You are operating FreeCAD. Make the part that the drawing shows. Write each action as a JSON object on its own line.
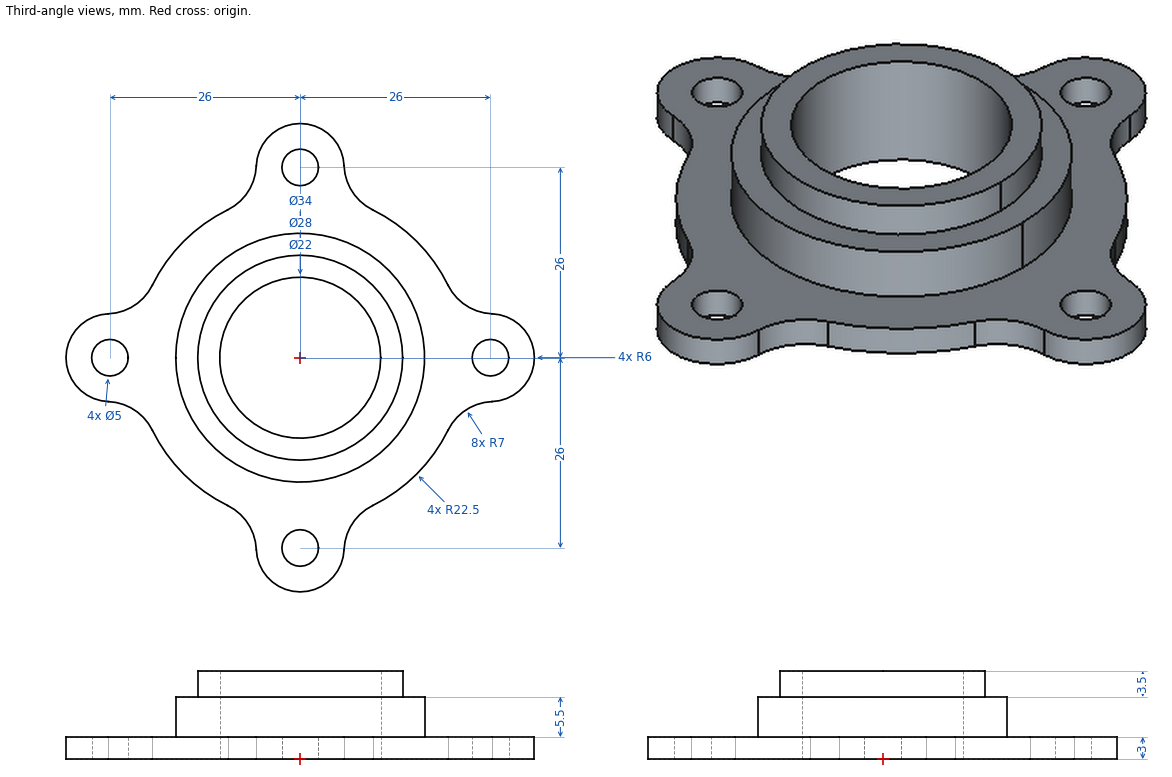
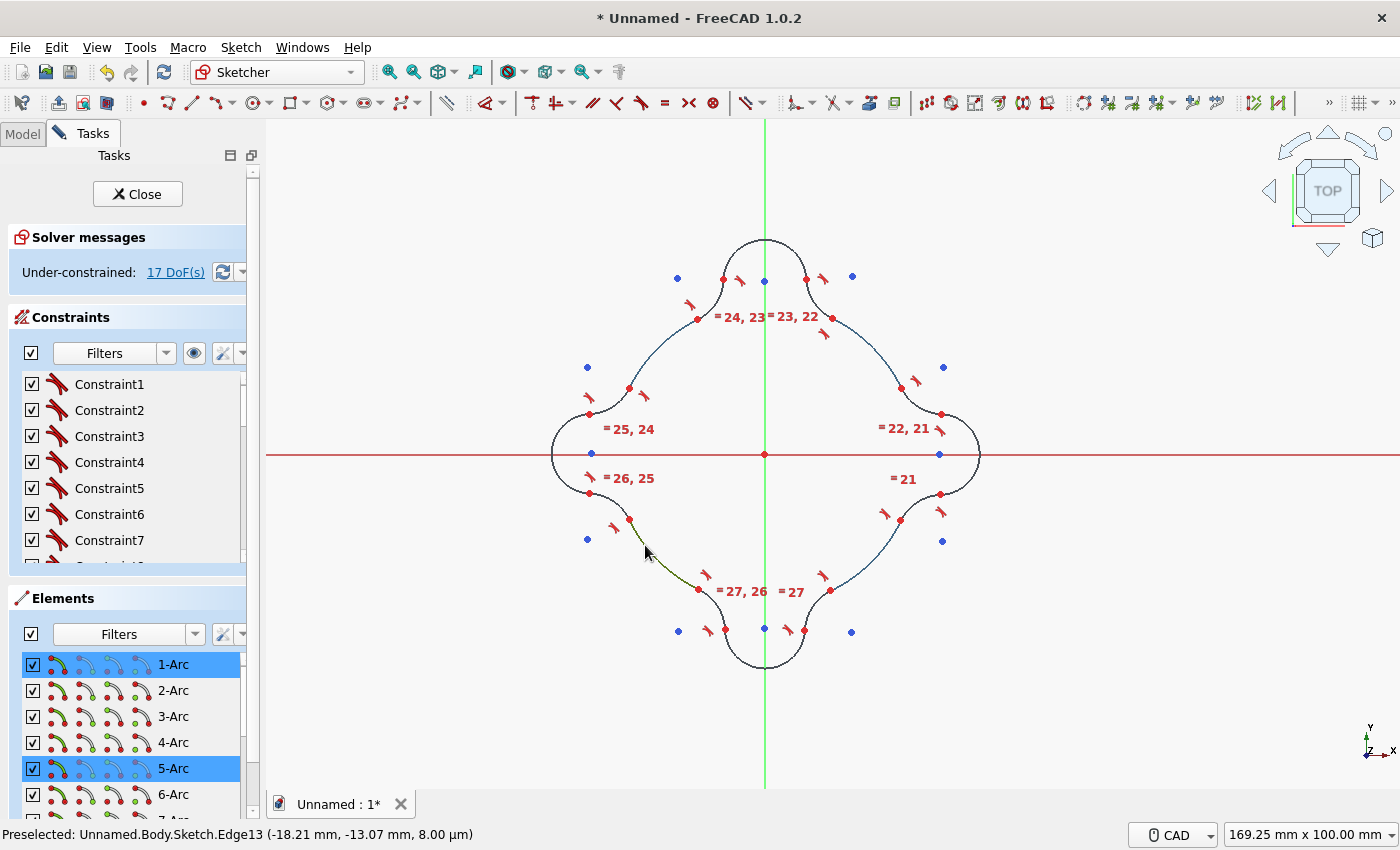
{"action": "left_click", "coordinate": [666, 104]}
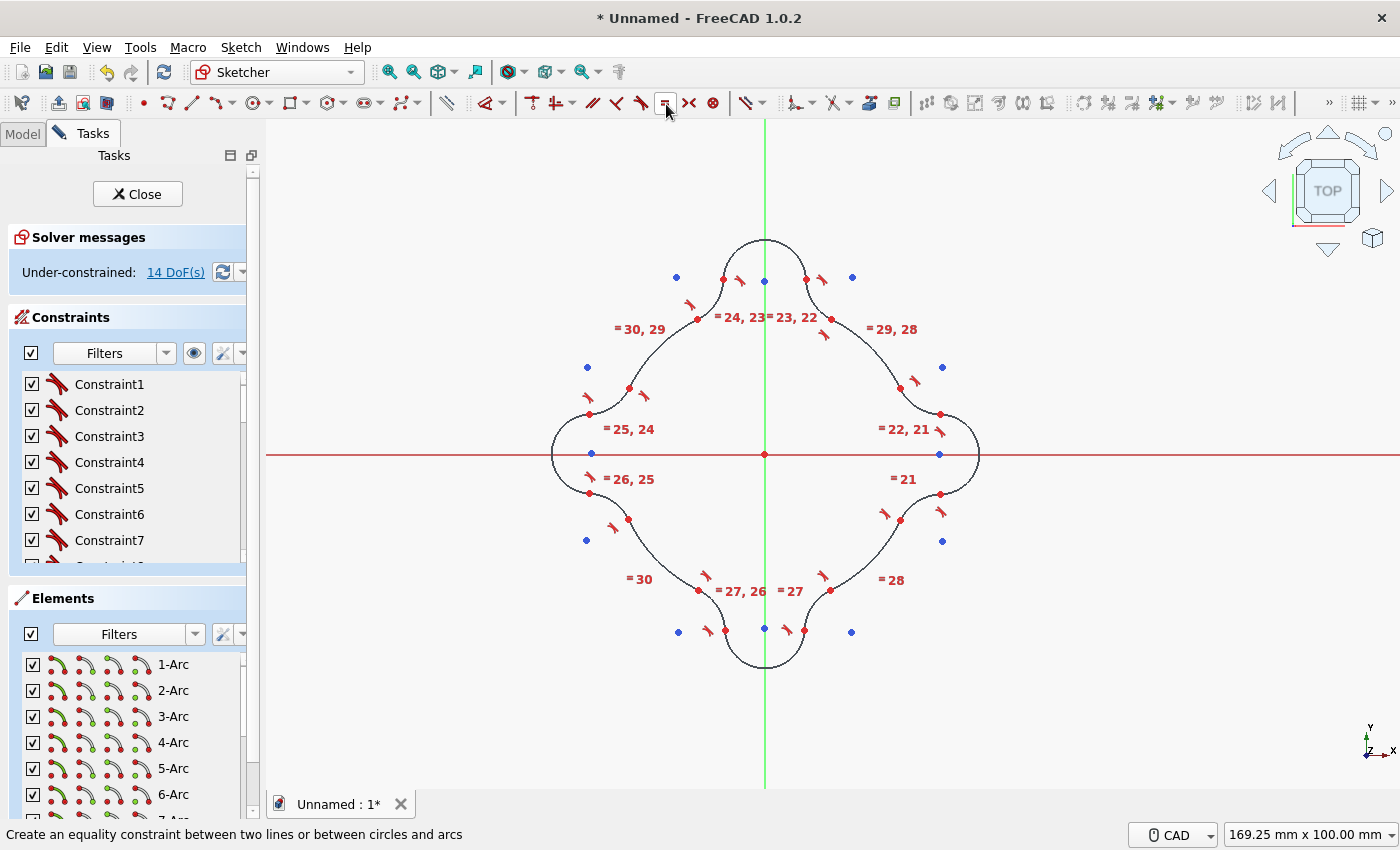
{"action": "left_click", "coordinate": [972, 478]}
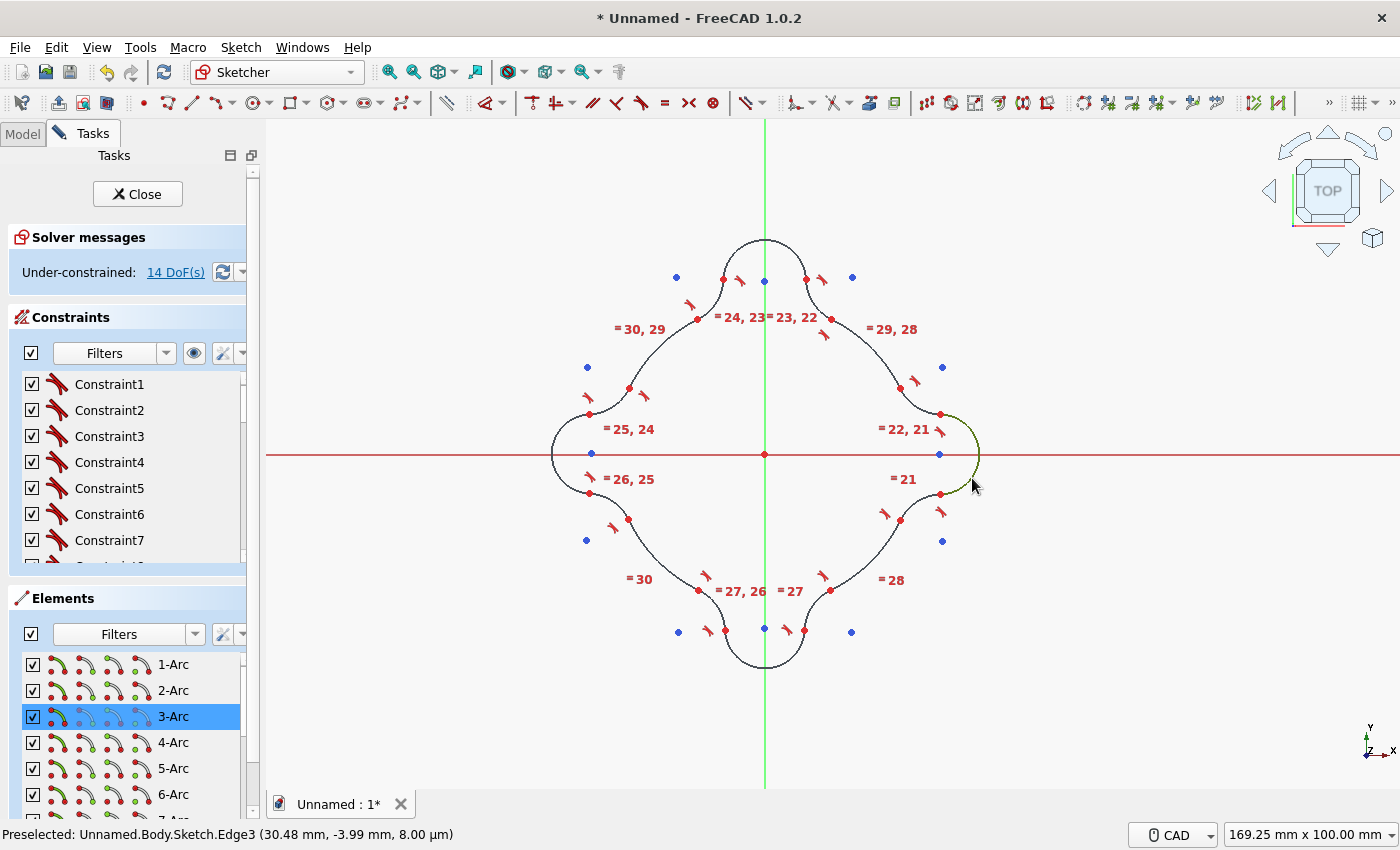
{"action": "left_click", "coordinate": [788, 248]}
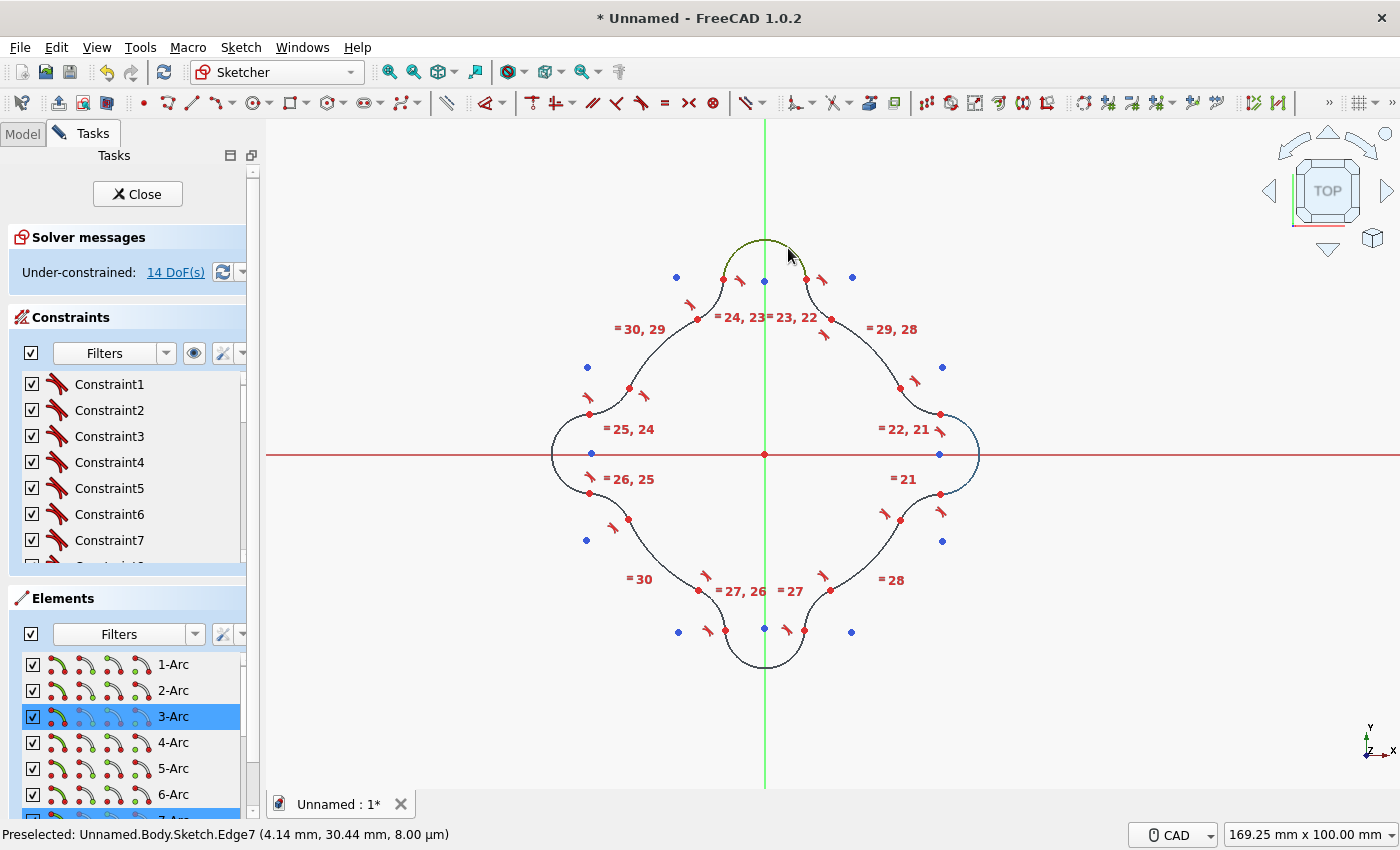
{"action": "left_click", "coordinate": [559, 431]}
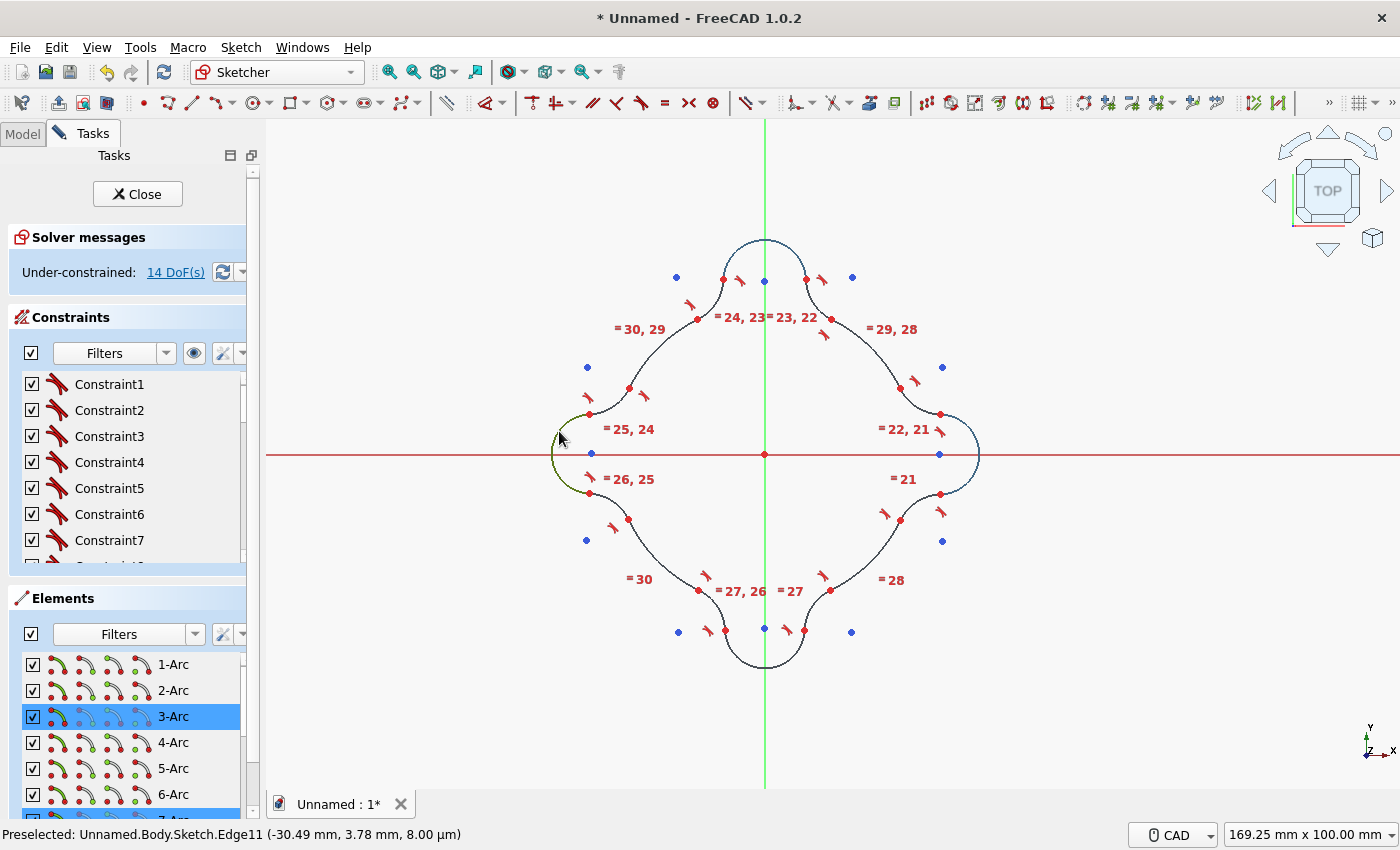
{"action": "left_click", "coordinate": [742, 661]}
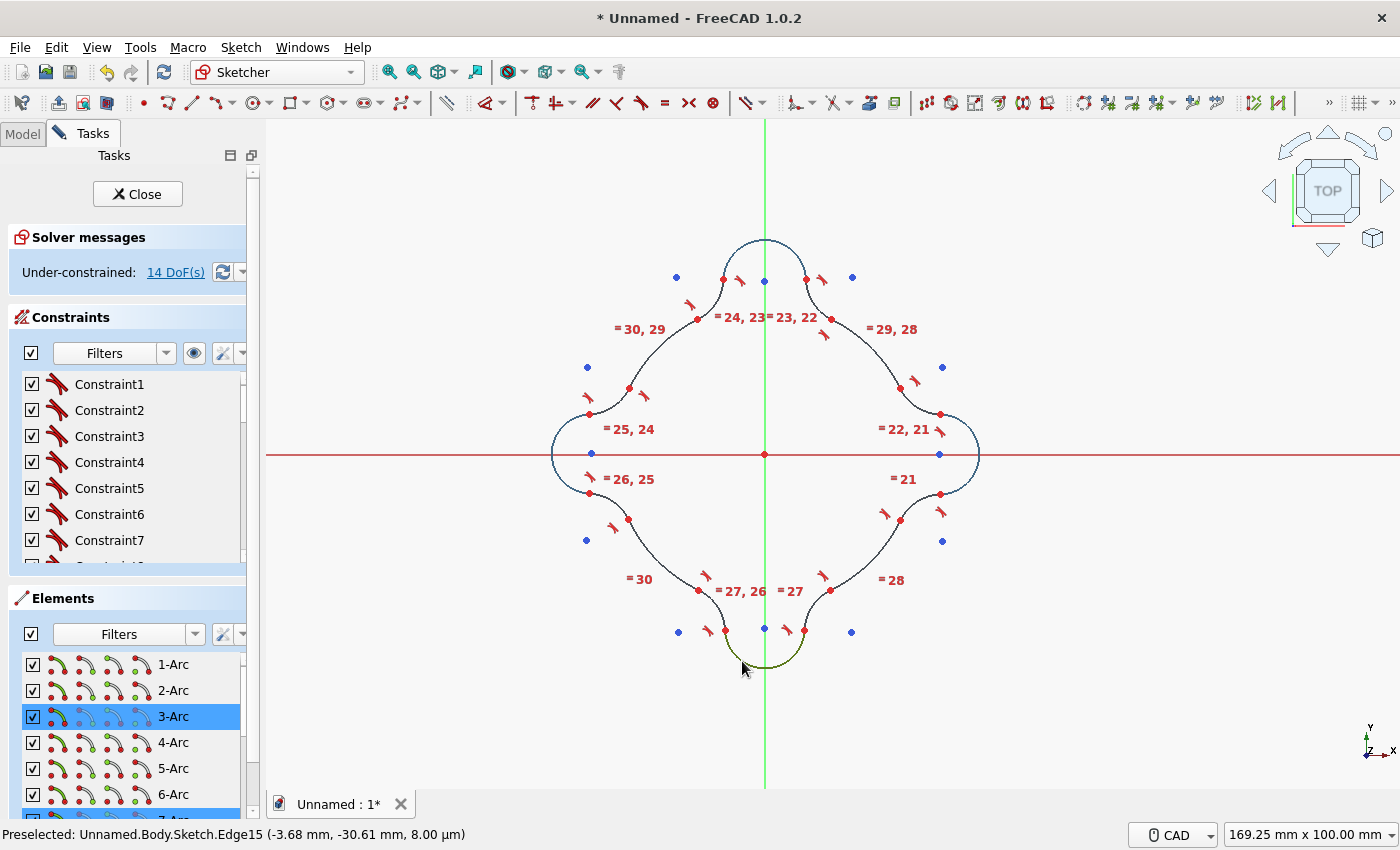
{"action": "left_click", "coordinate": [666, 104]}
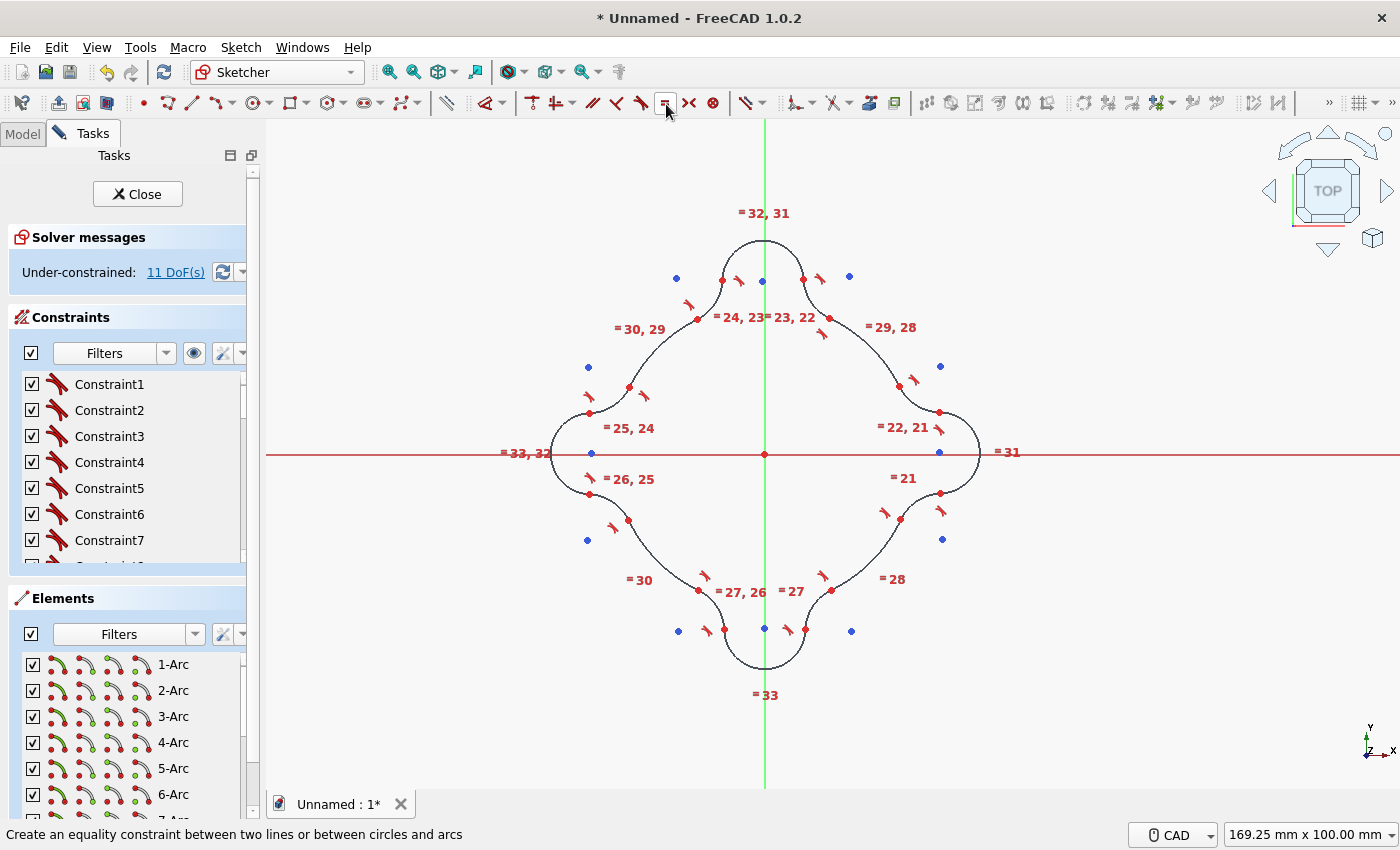
{"action": "left_click", "coordinate": [939, 453]}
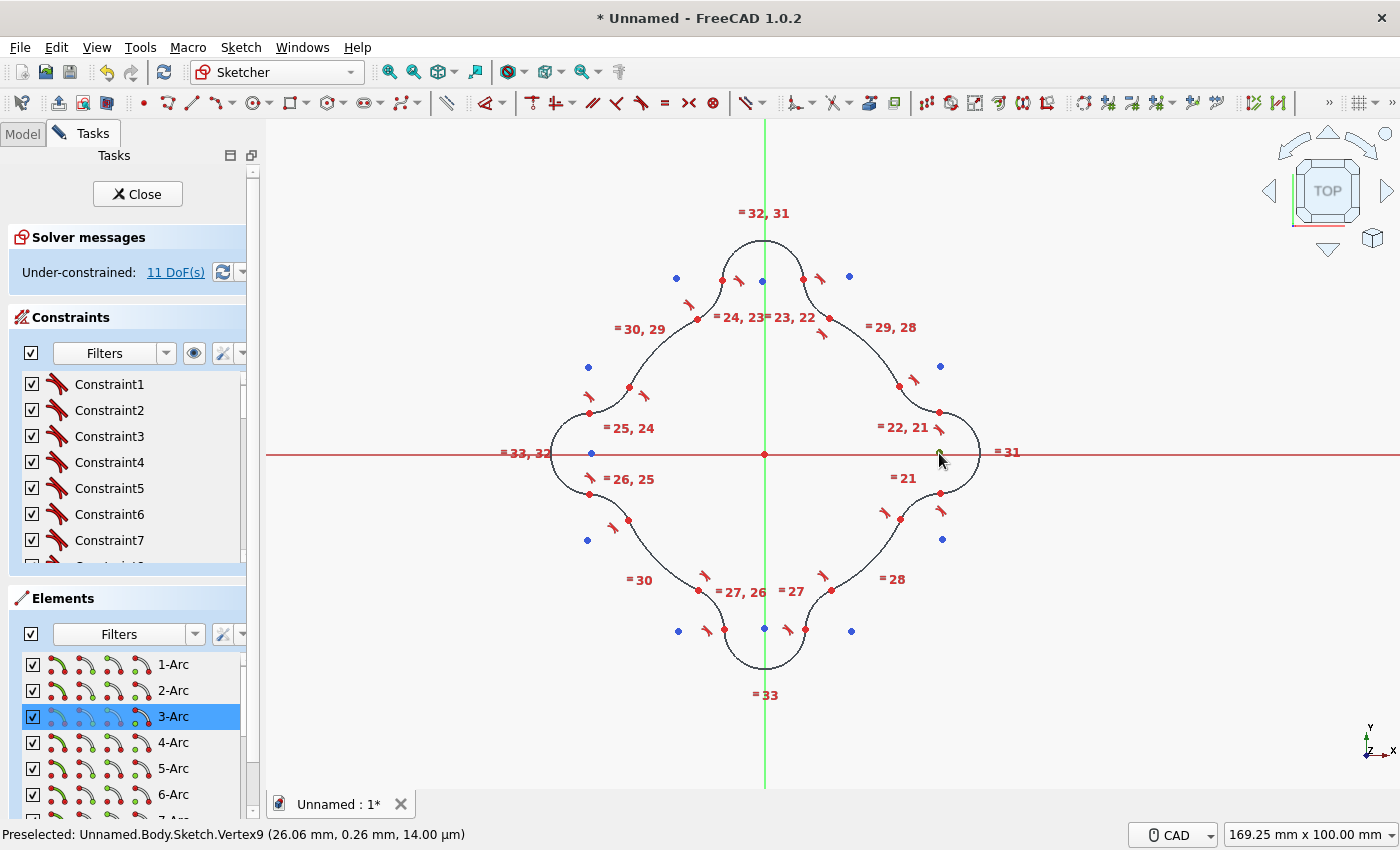
{"action": "left_click", "coordinate": [361, 455]}